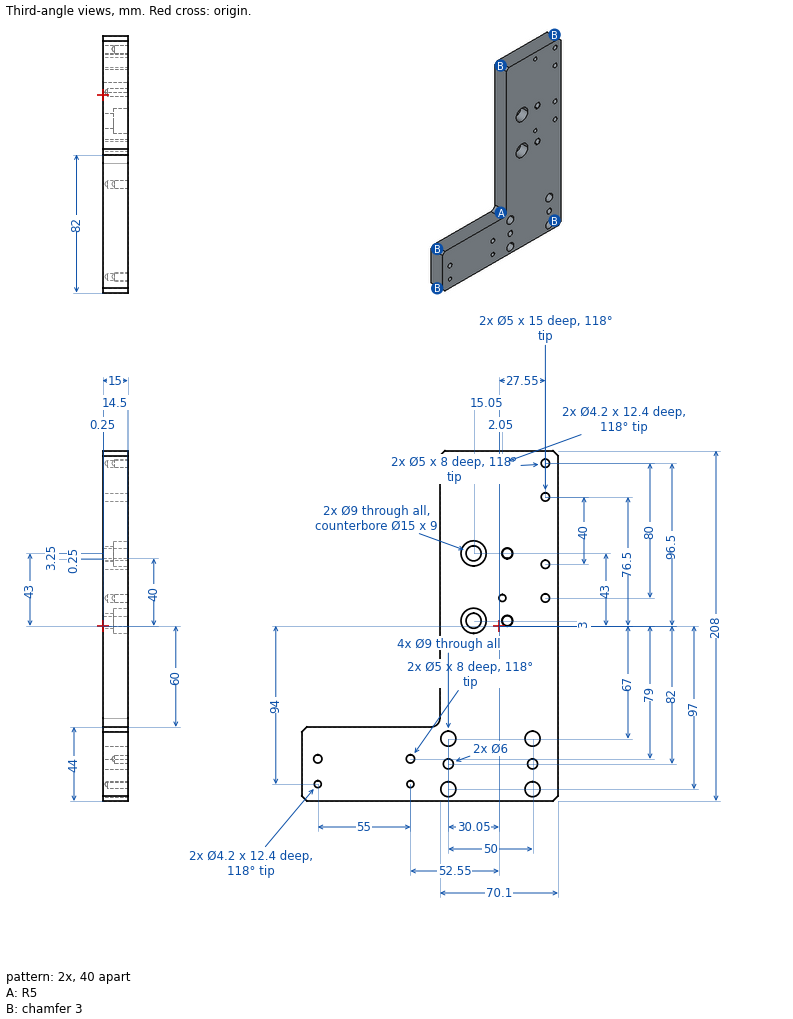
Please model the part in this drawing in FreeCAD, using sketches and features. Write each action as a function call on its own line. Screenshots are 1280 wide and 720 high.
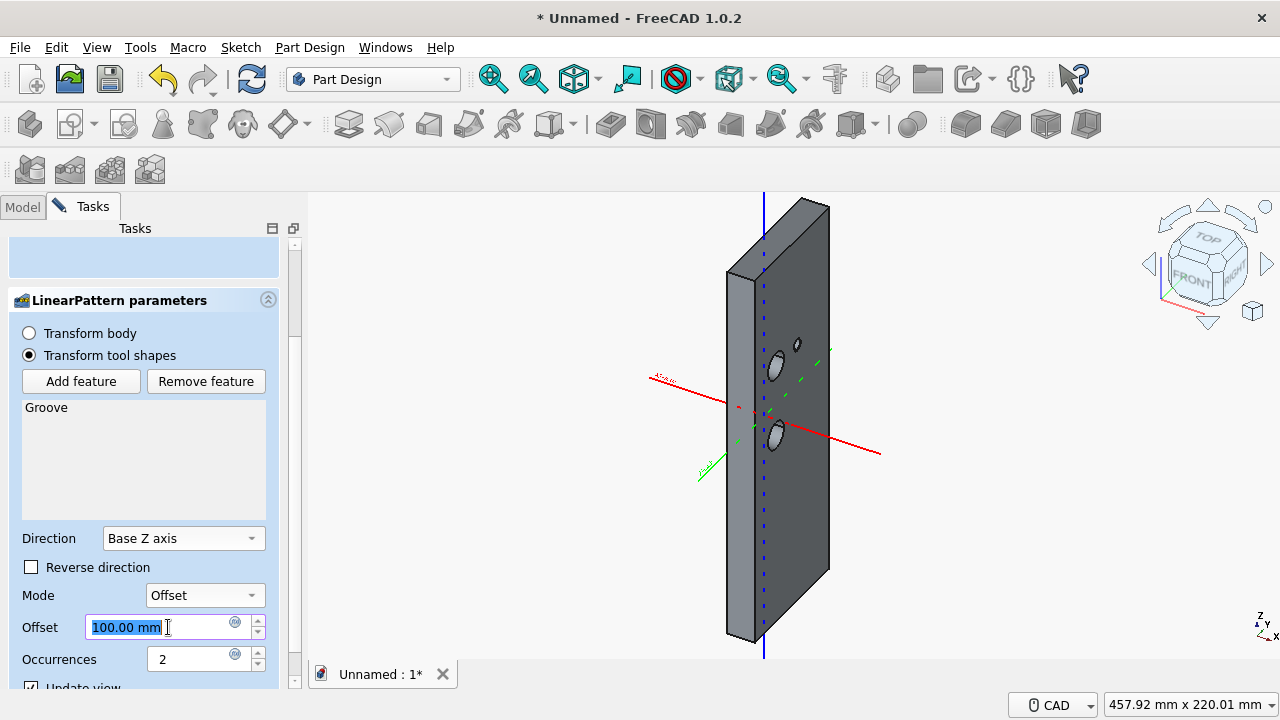
text(40)
key(Tab)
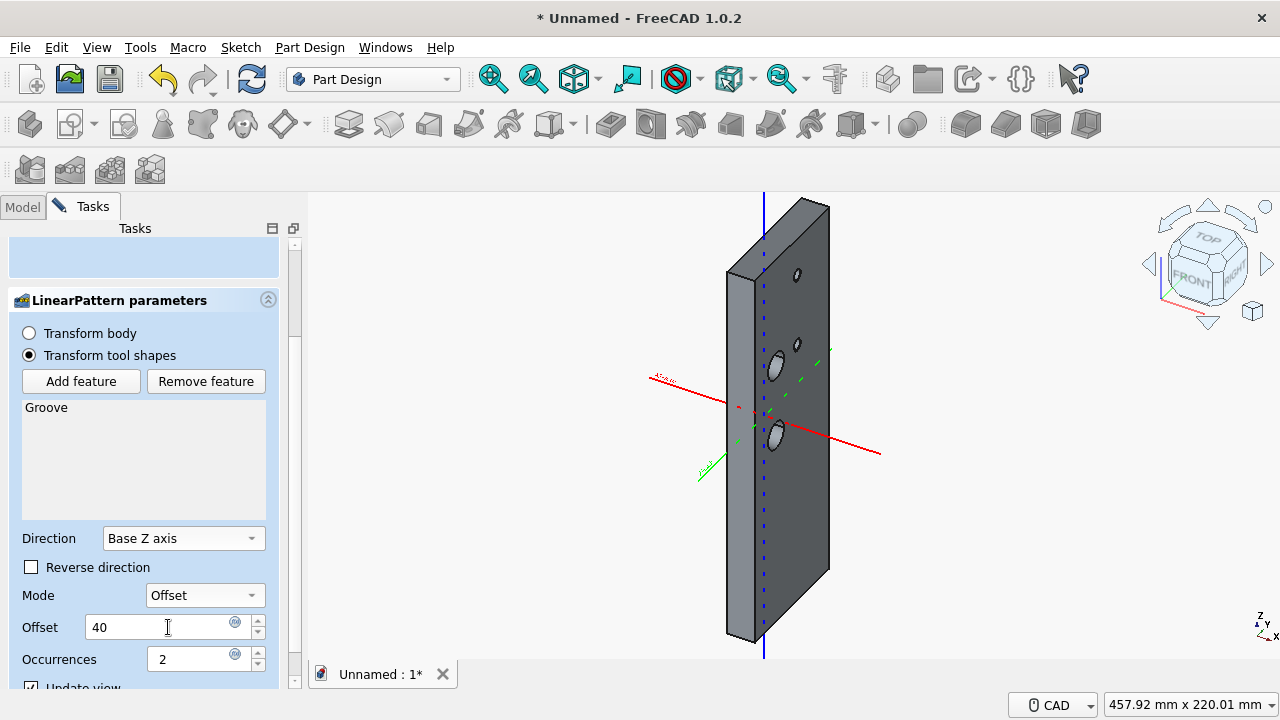
triple_click(198, 659)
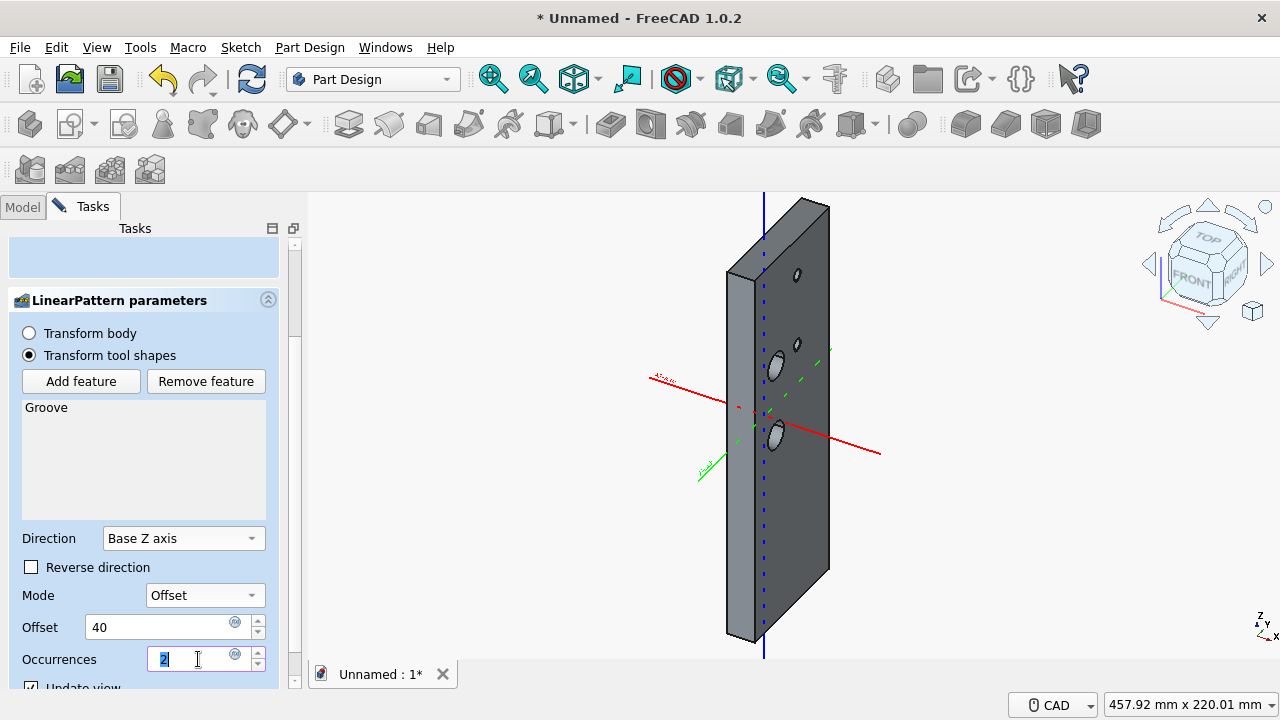
text(2)
key(Tab)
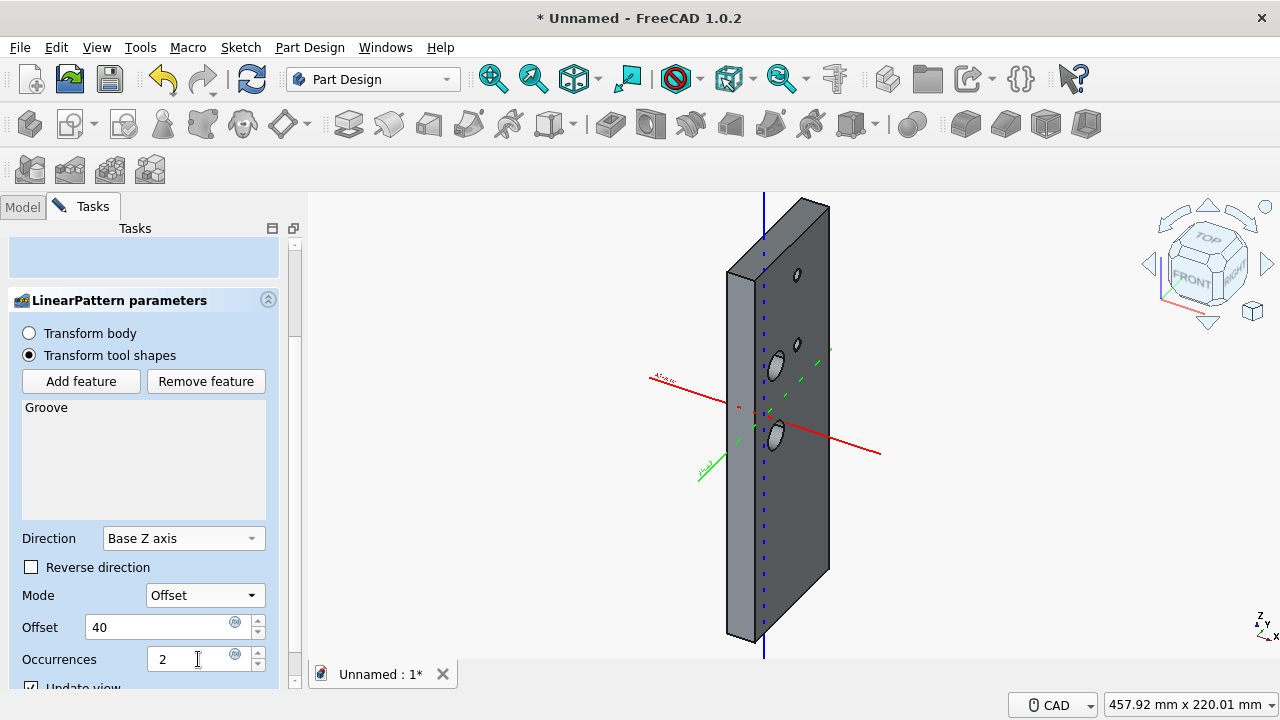
click(30, 567)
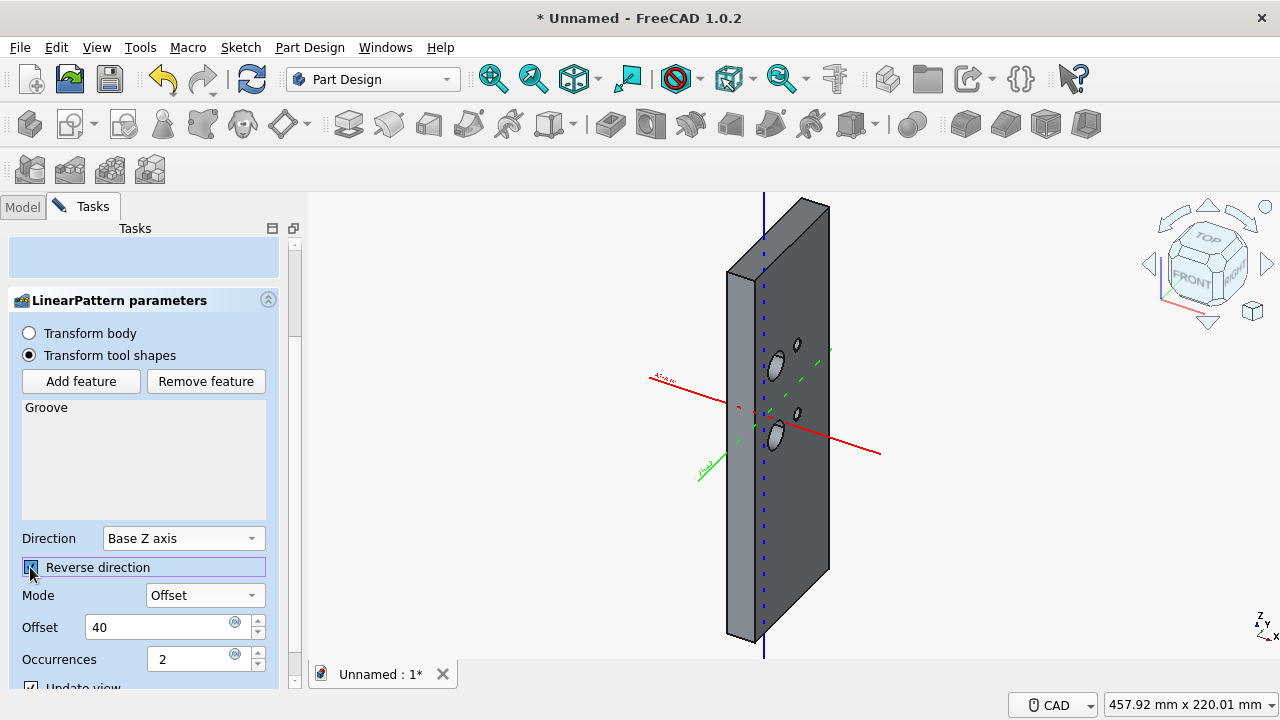
scroll(295, 463, up, 3)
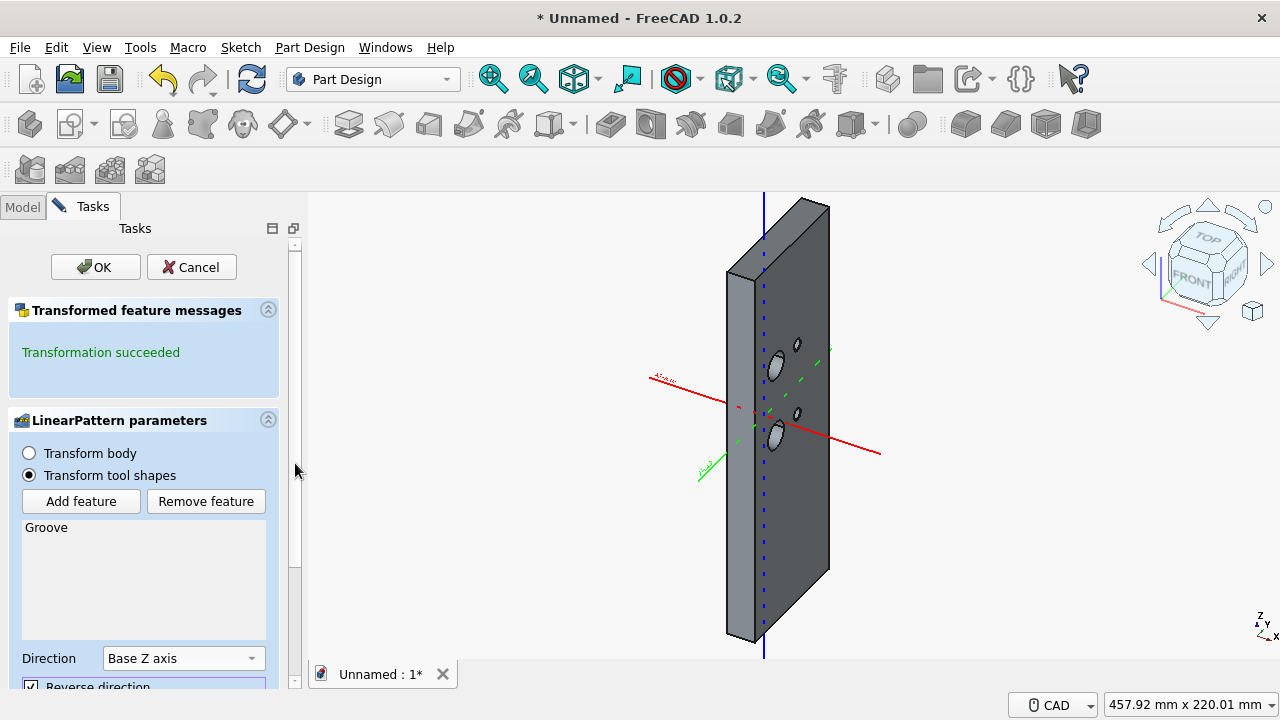
click(96, 267)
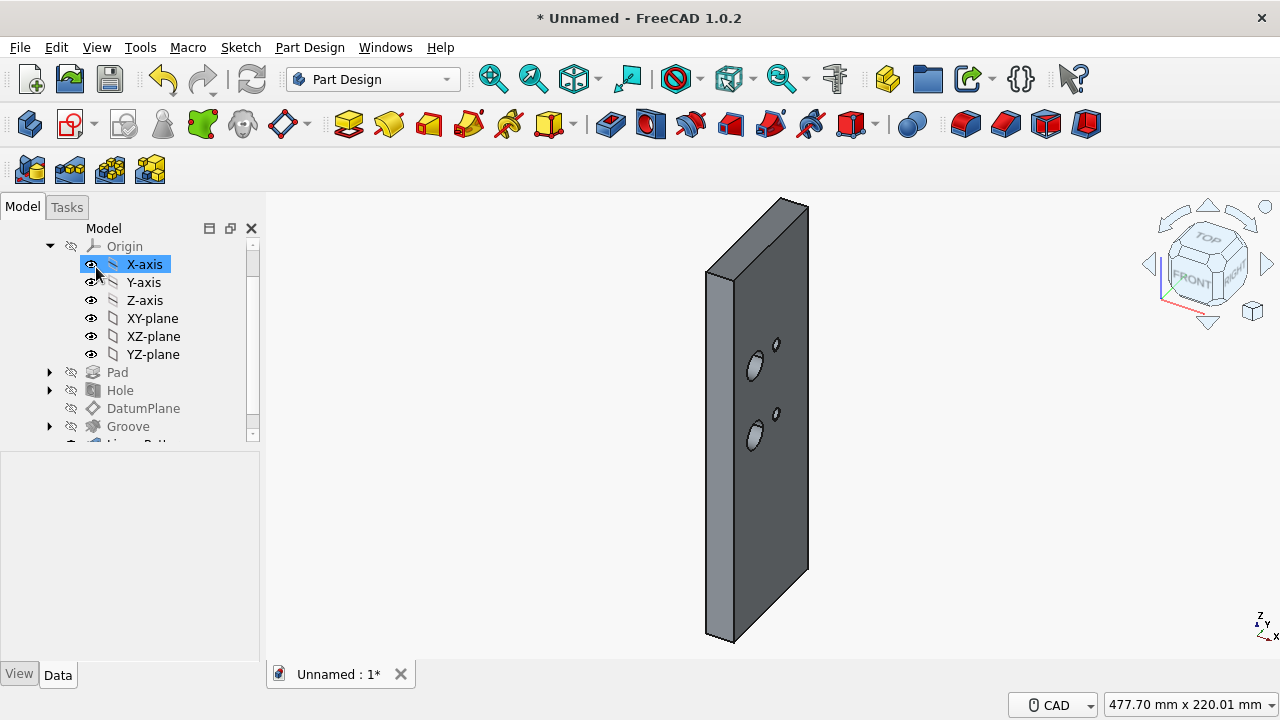
click(720, 611)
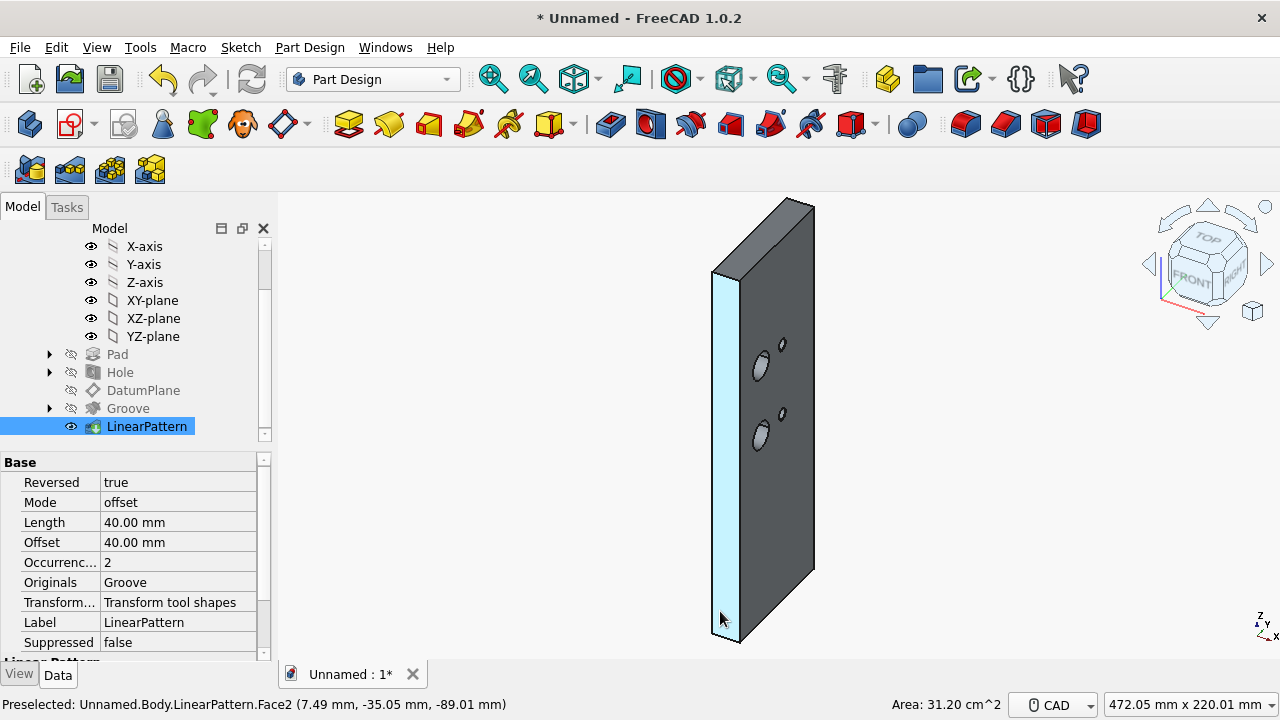
click(70, 124)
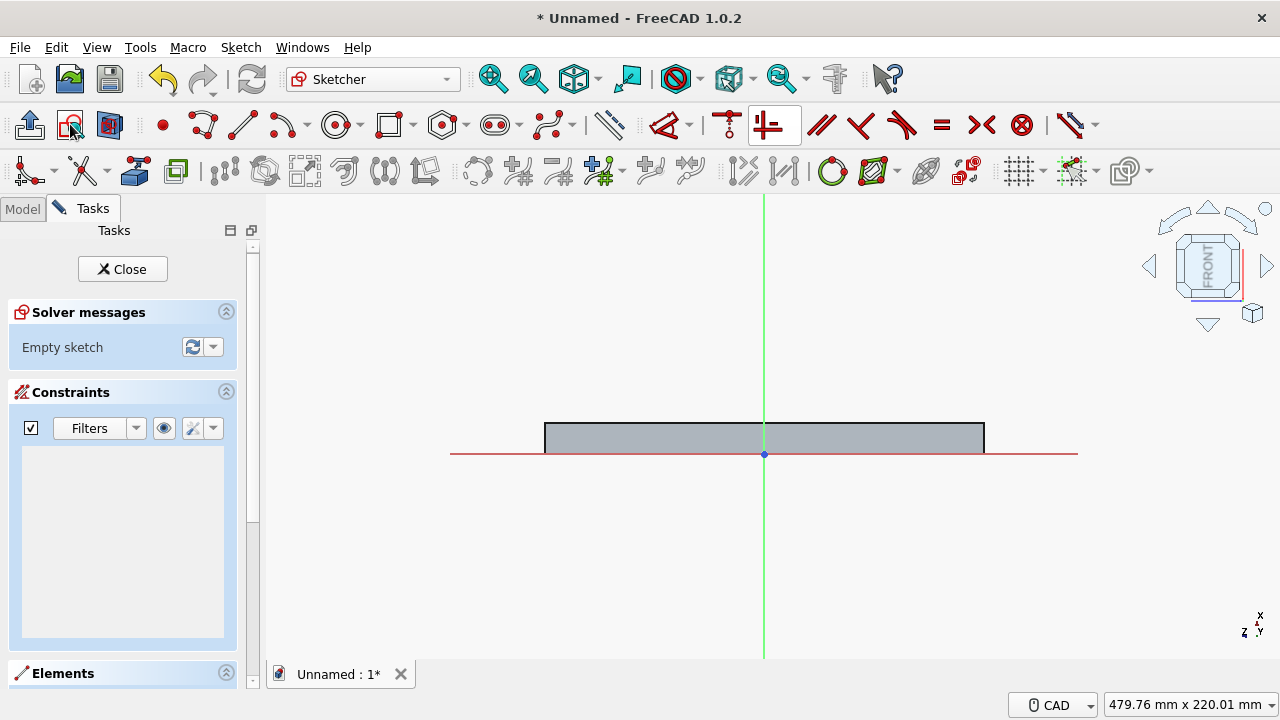
scroll(973, 446, up, 5)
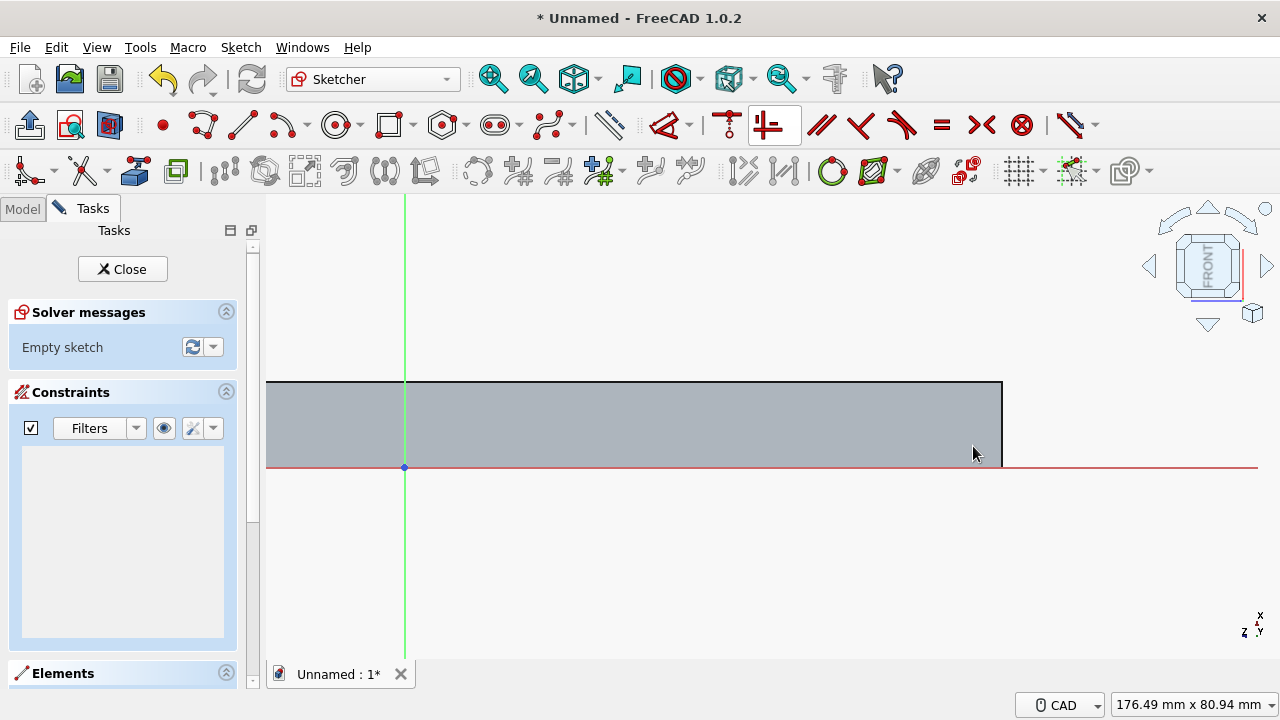
click(390, 126)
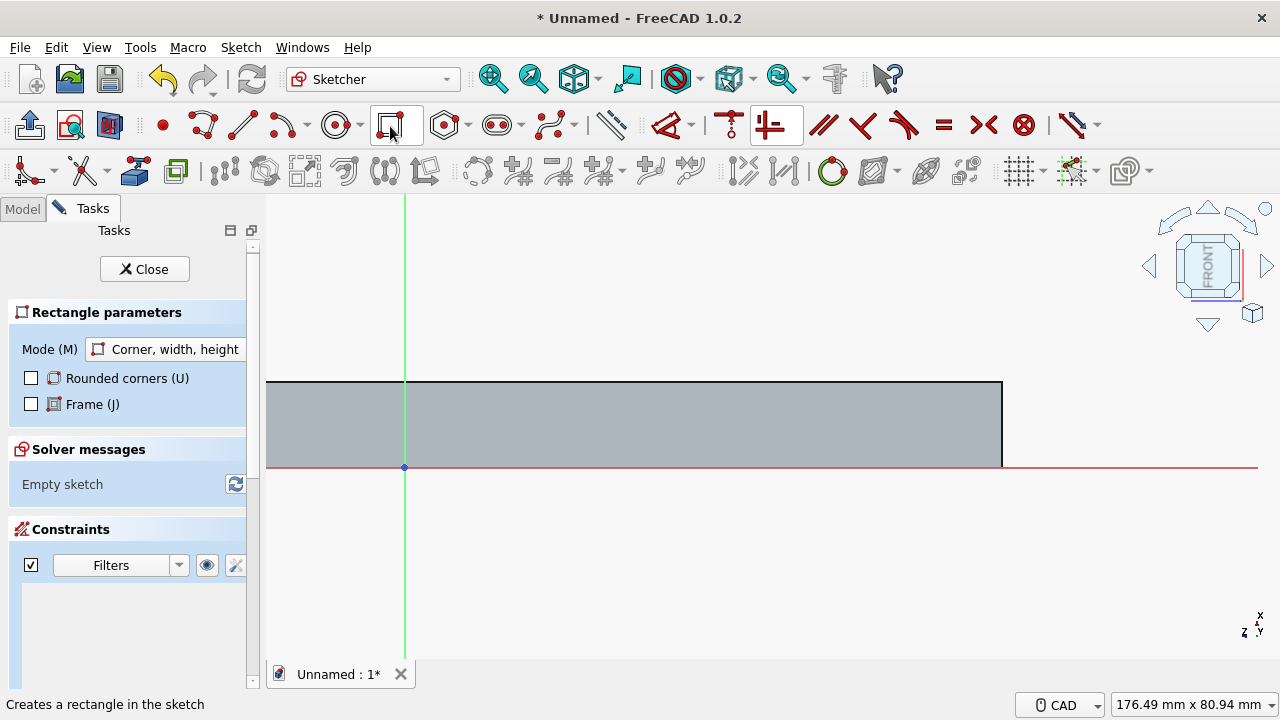
click(750, 382)
click(1002, 468)
key(Escape)